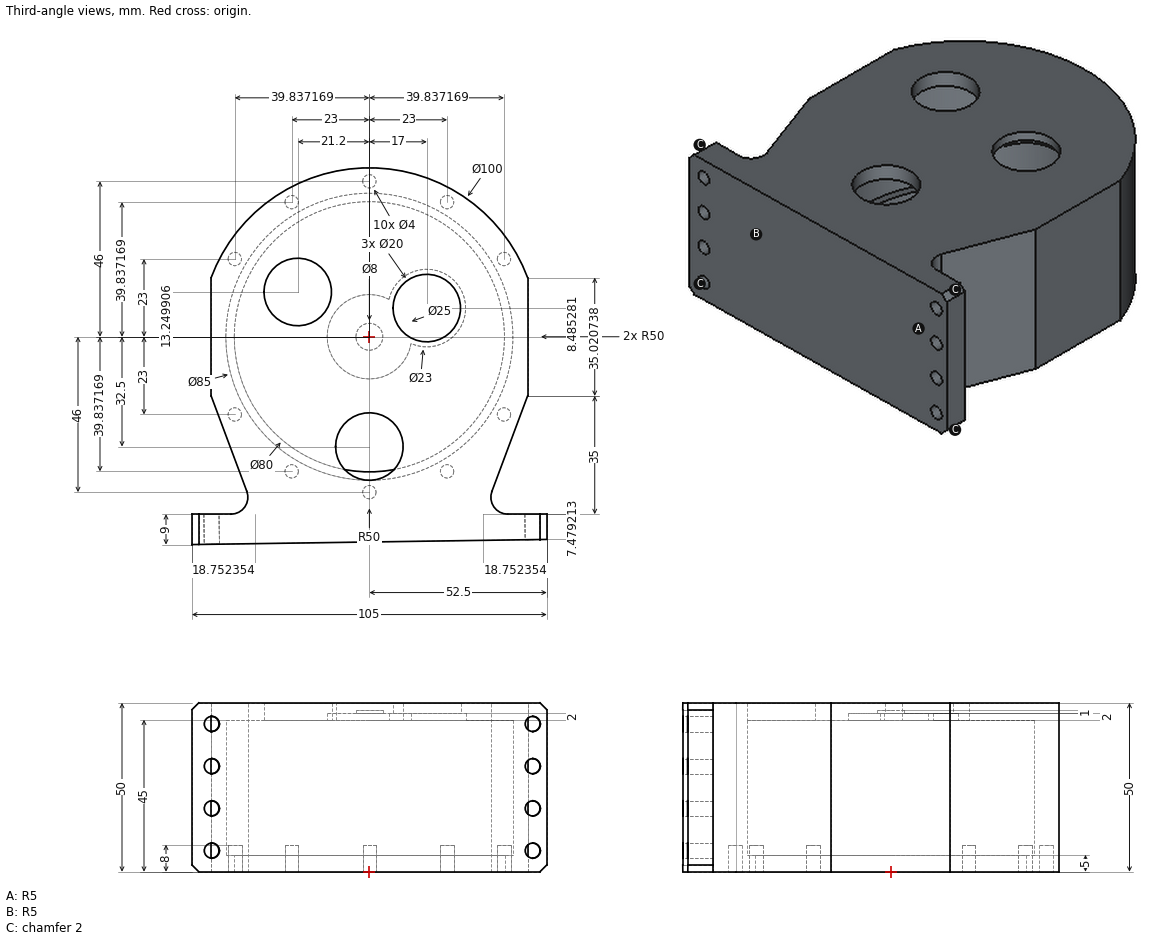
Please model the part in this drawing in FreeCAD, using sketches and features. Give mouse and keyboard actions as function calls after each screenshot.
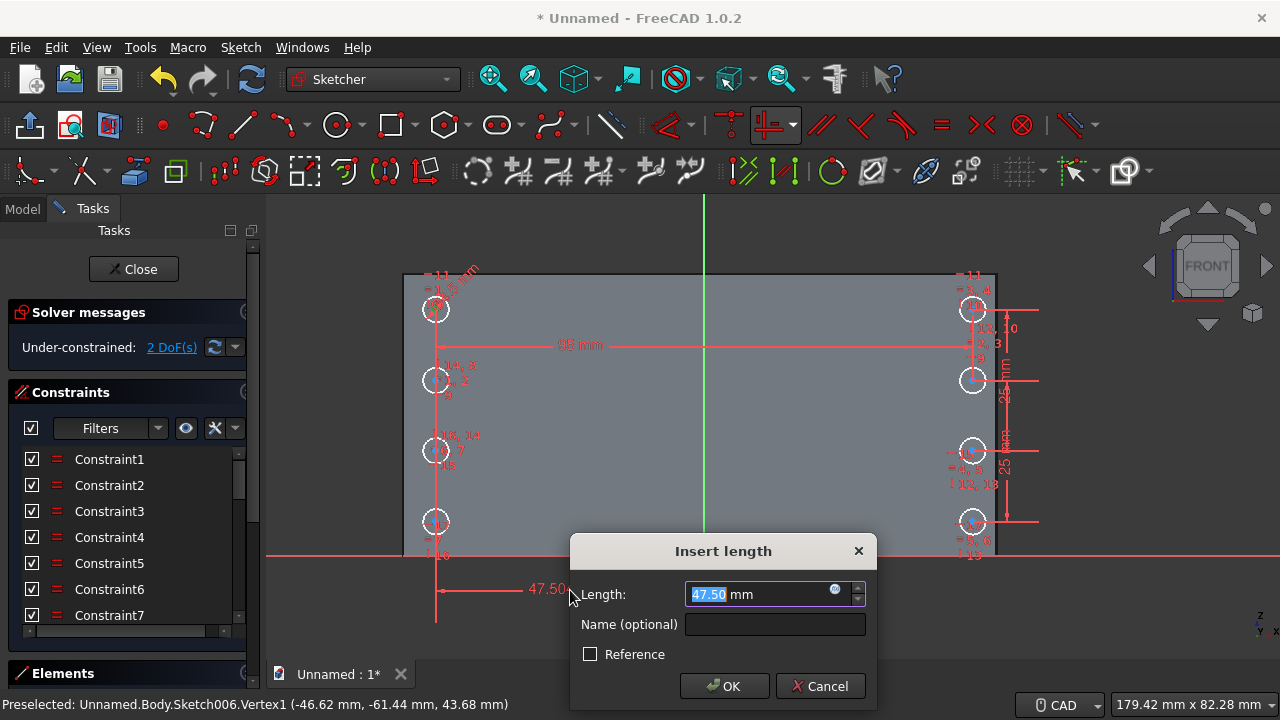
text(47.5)
key(Return)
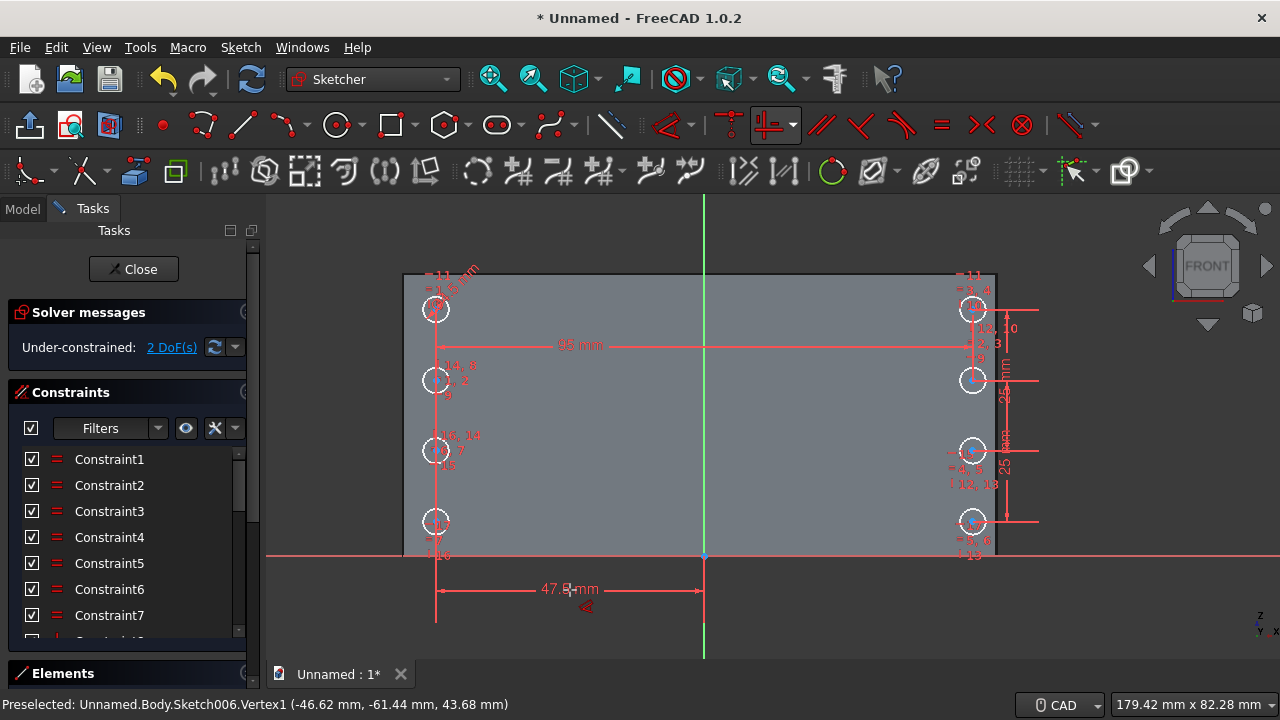
click(973, 522)
click(1007, 539)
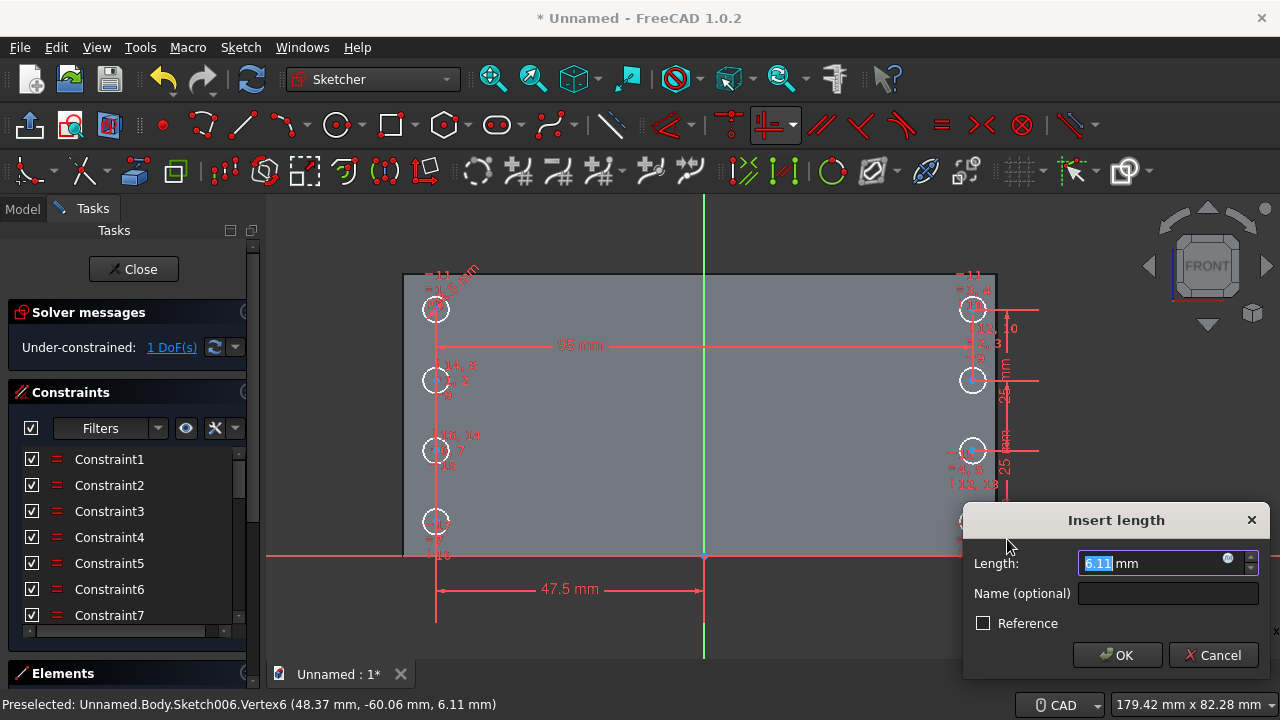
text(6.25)
key(Return)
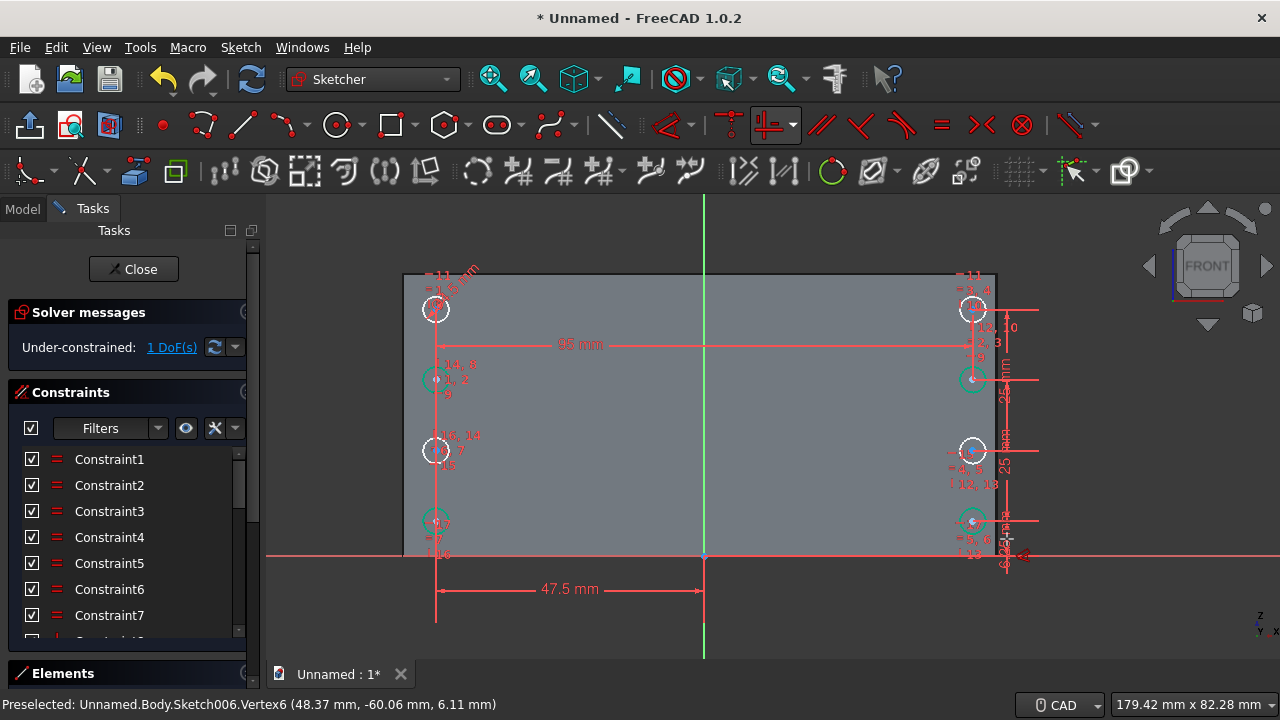
click(436, 310)
click(402, 433)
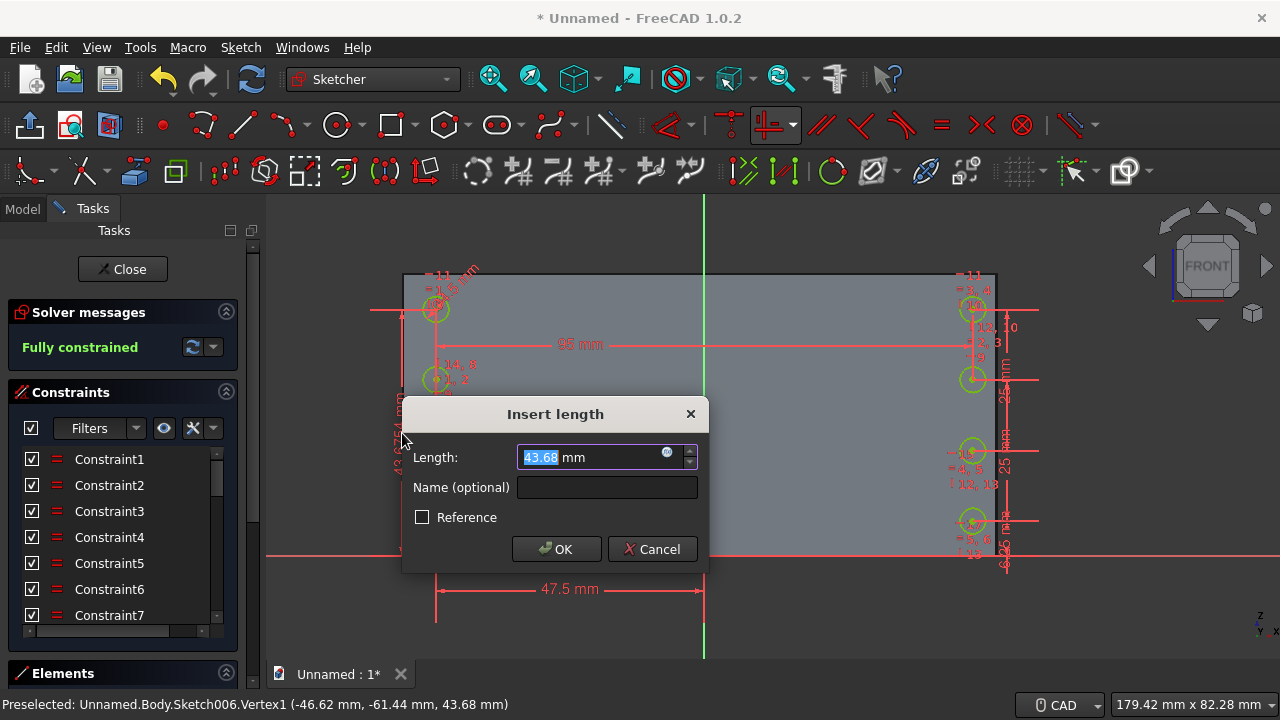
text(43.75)
key(Return)
key(Escape)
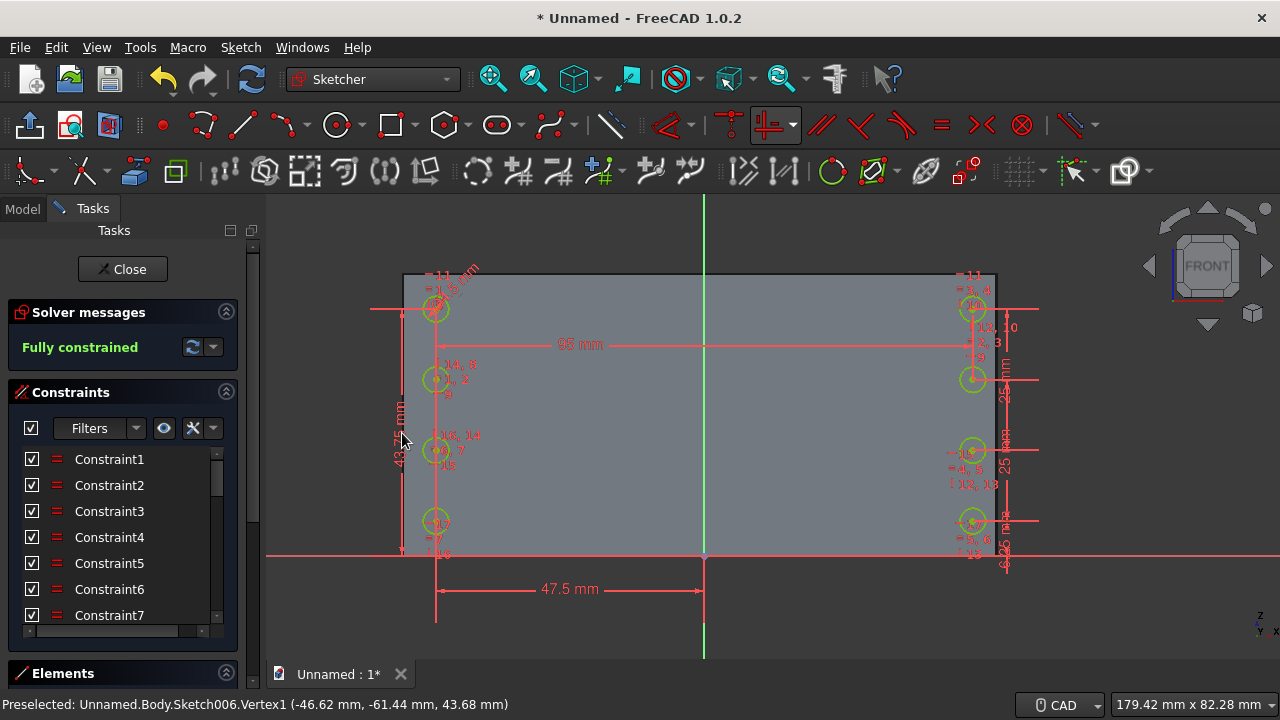
click(123, 269)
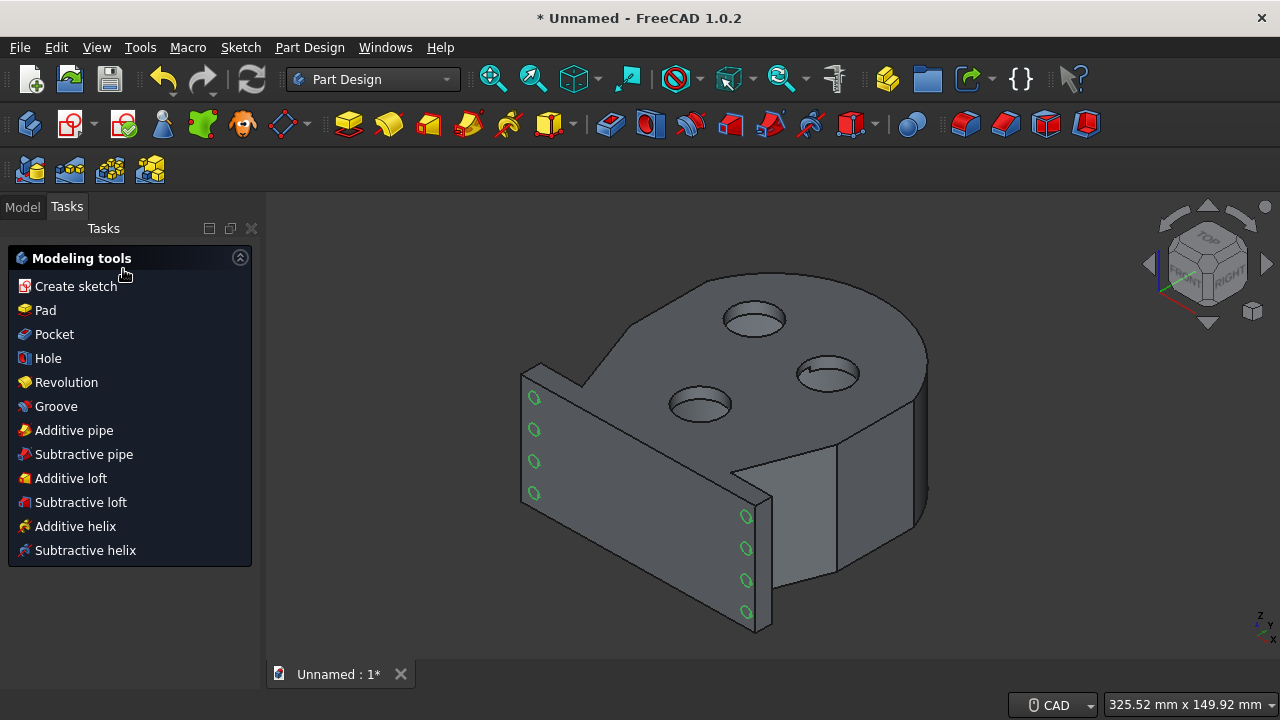
click(612, 124)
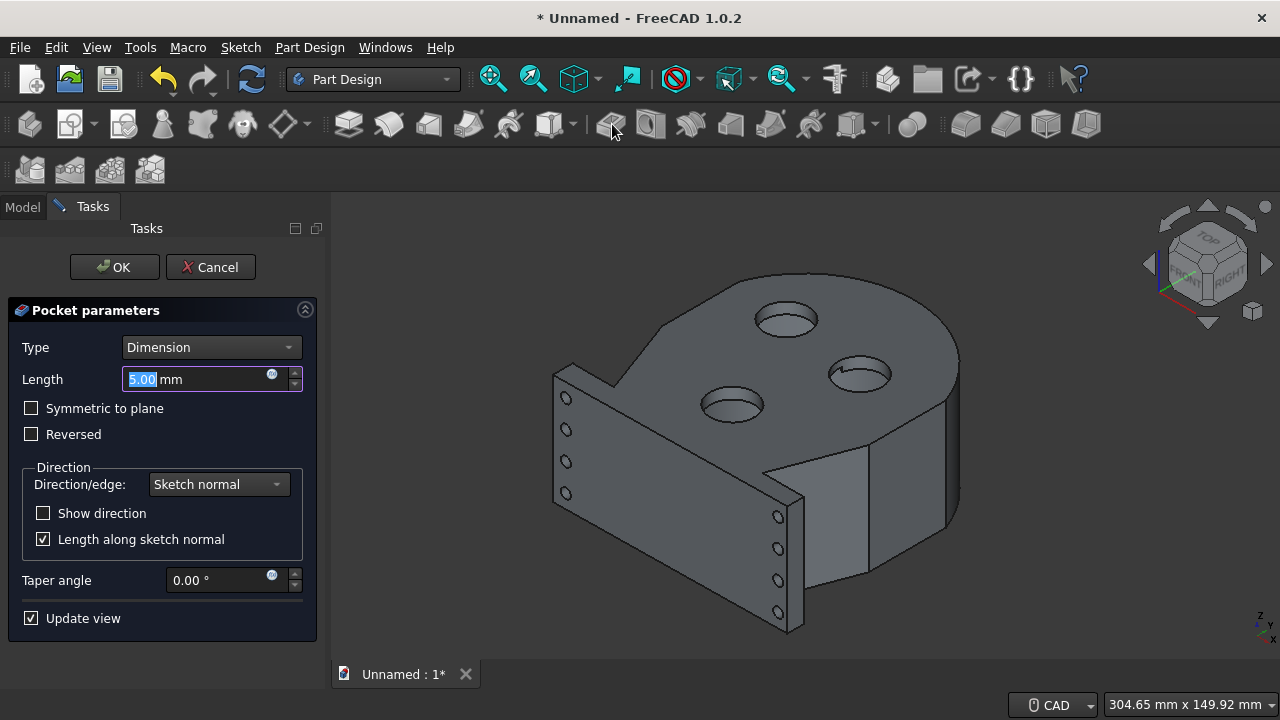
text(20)
key(Tab)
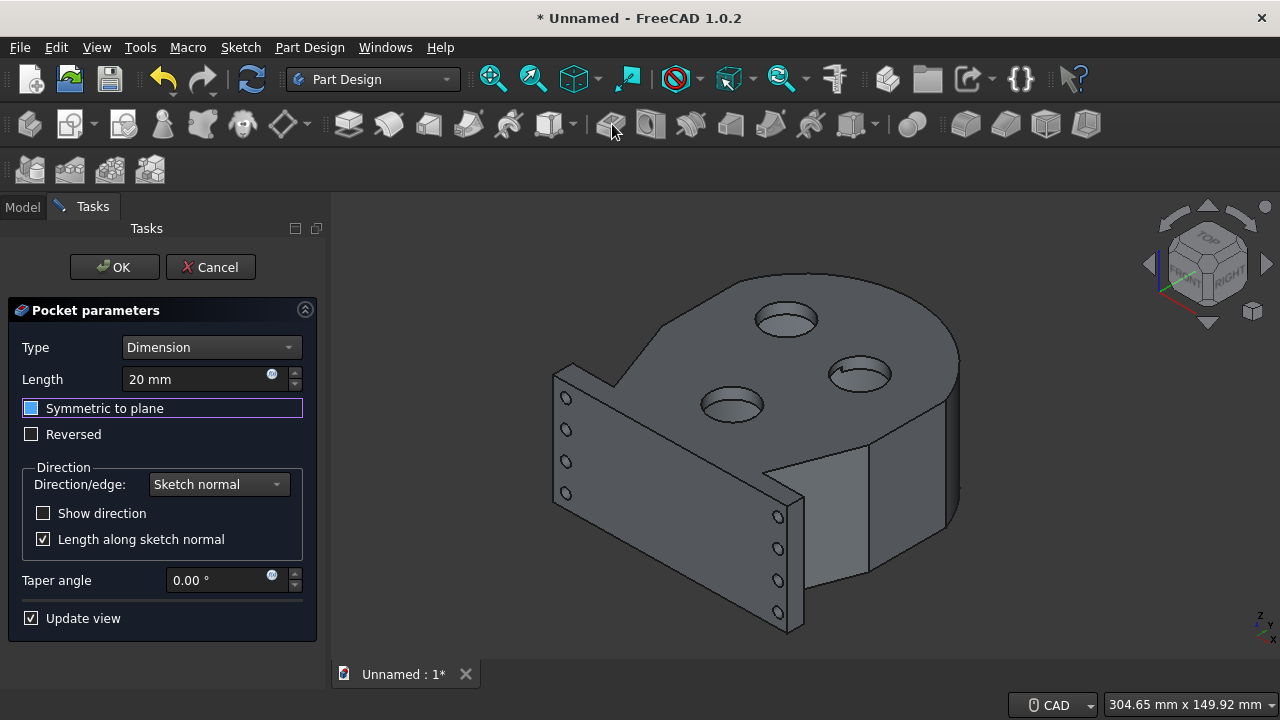
click(115, 267)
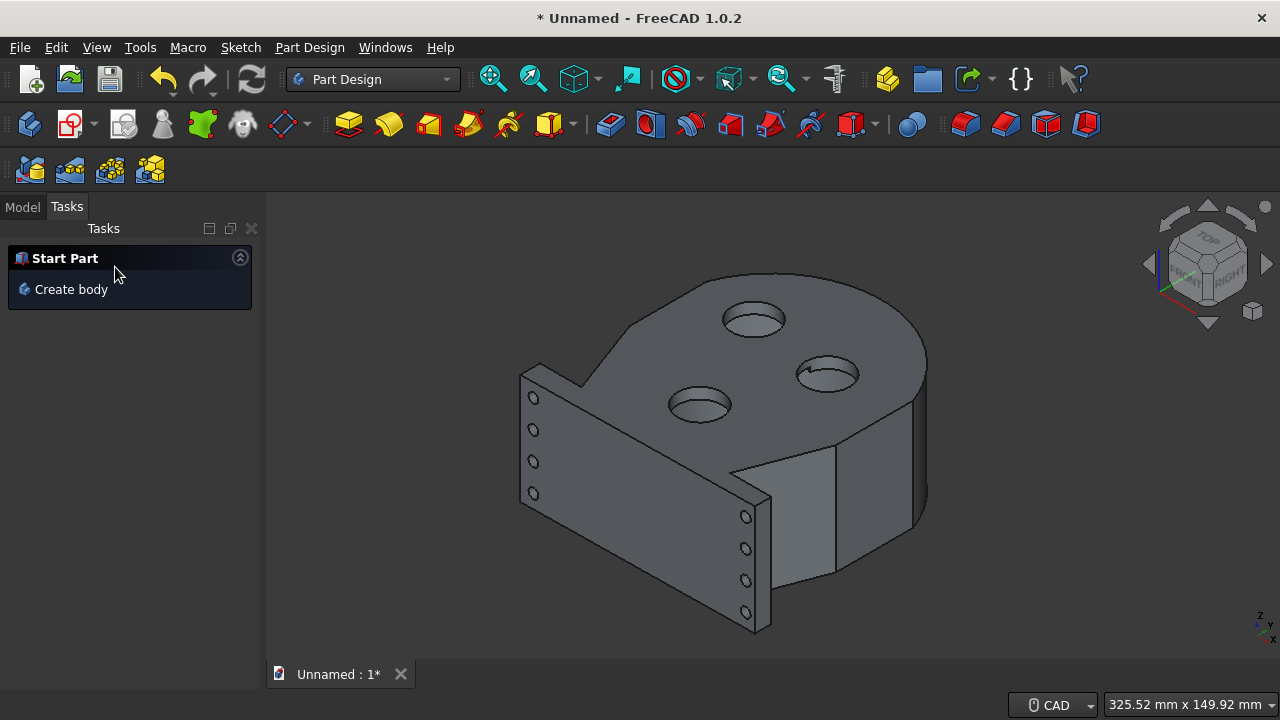
key(2)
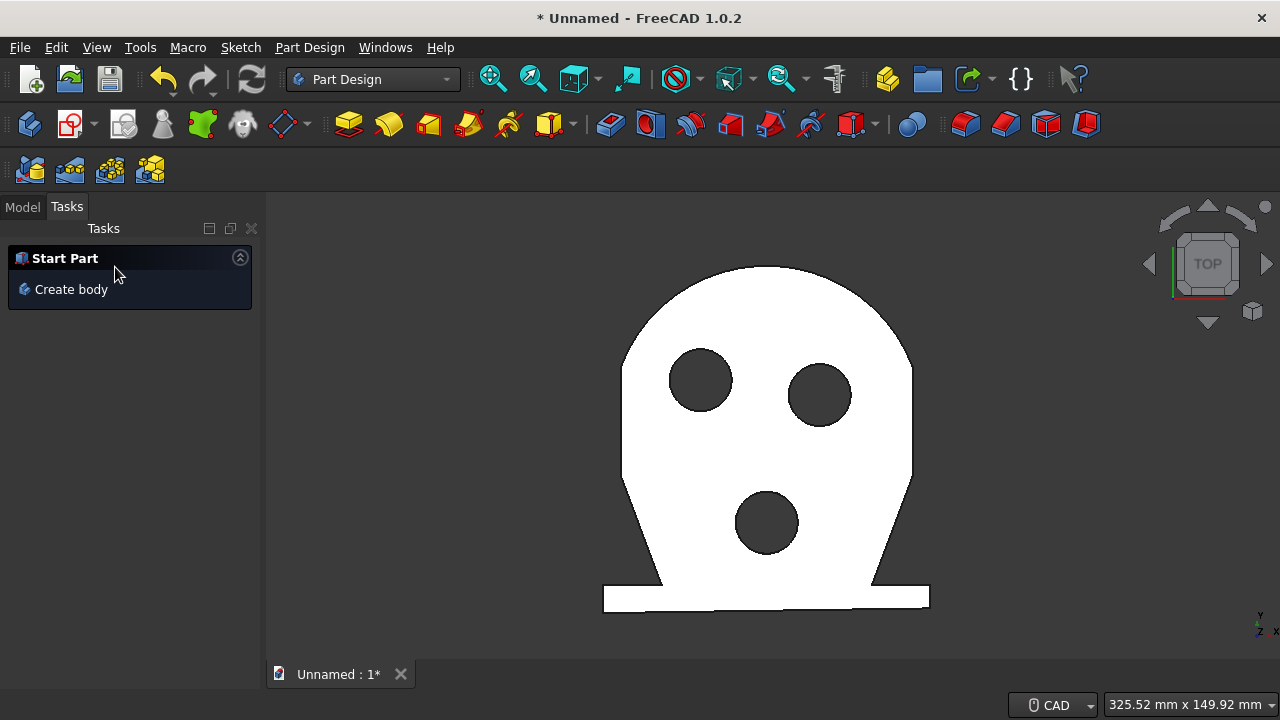
key(0)